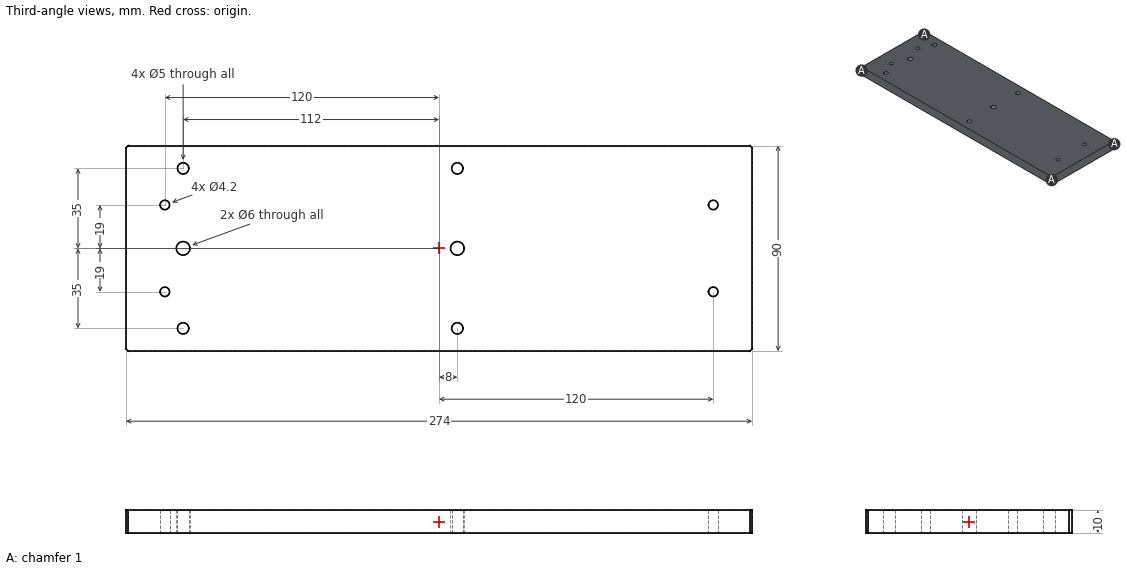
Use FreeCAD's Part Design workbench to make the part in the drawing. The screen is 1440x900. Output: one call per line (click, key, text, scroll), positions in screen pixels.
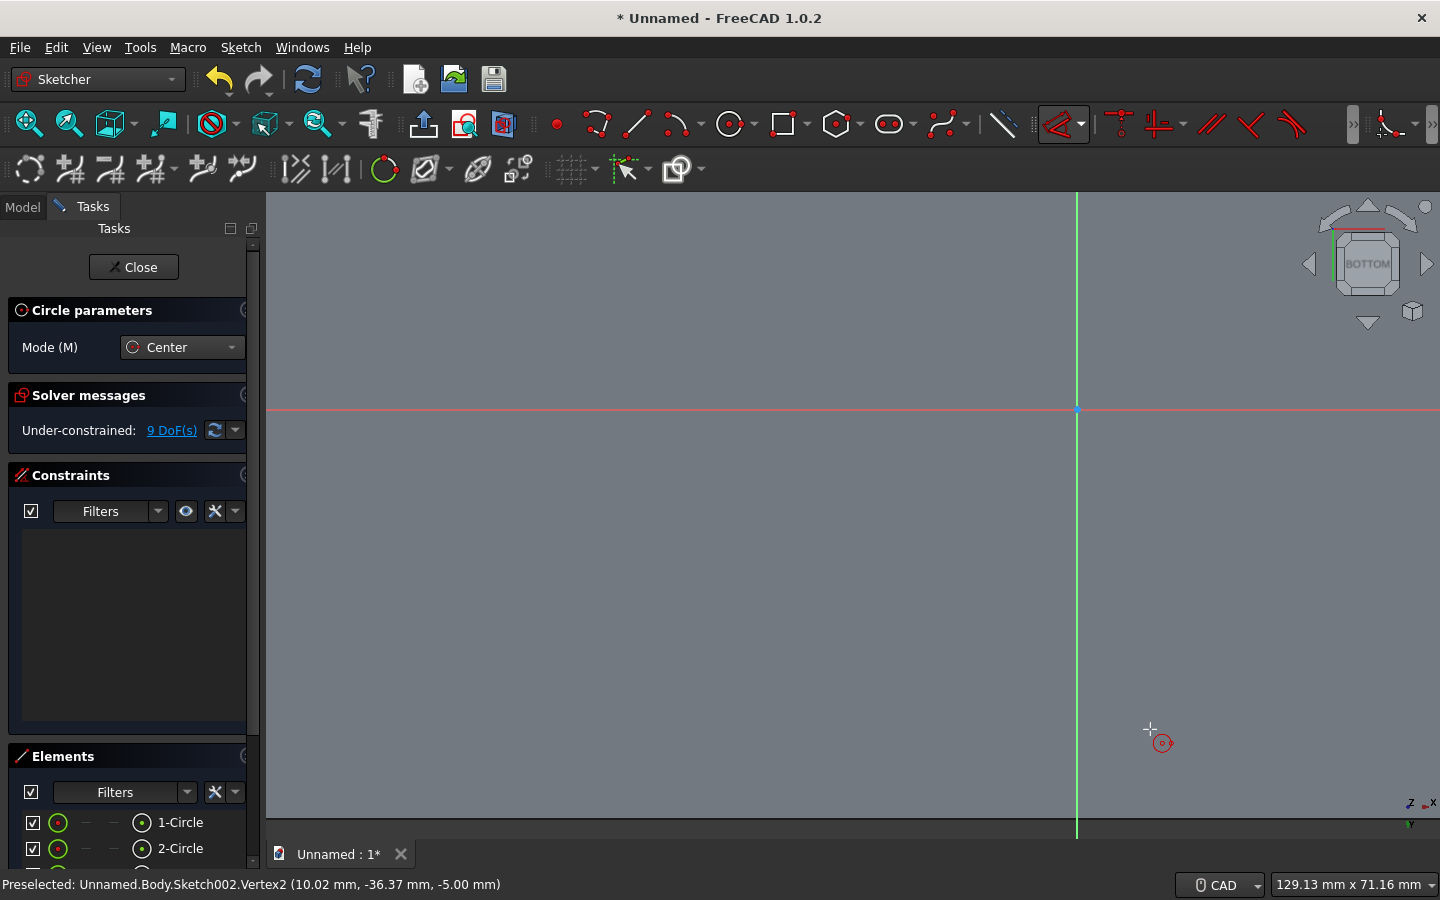
click(1150, 728)
click(1166, 712)
key(Escape)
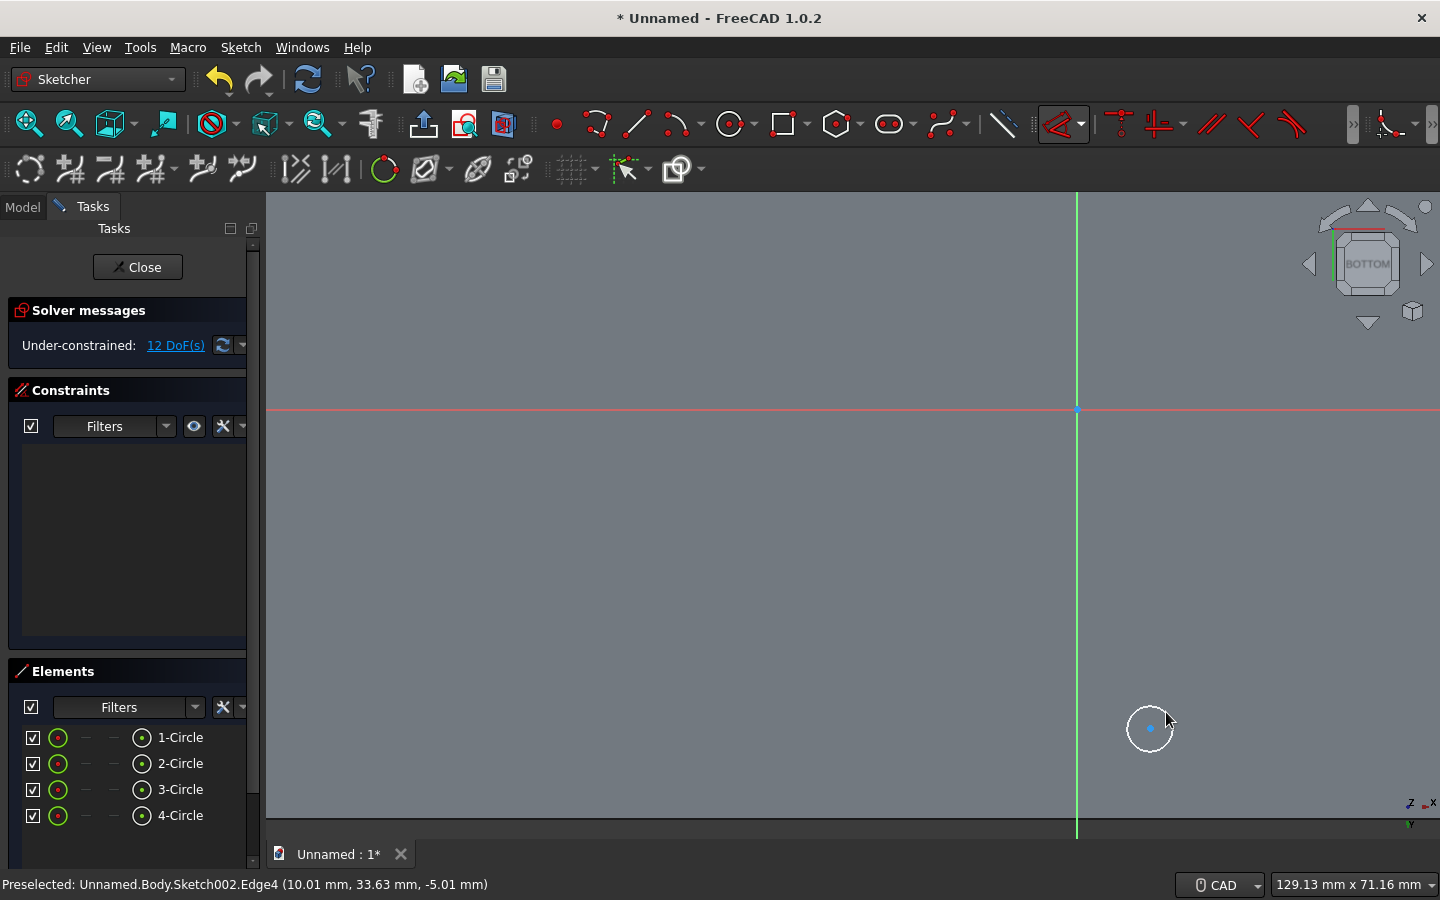
scroll(1150, 730, down, 2)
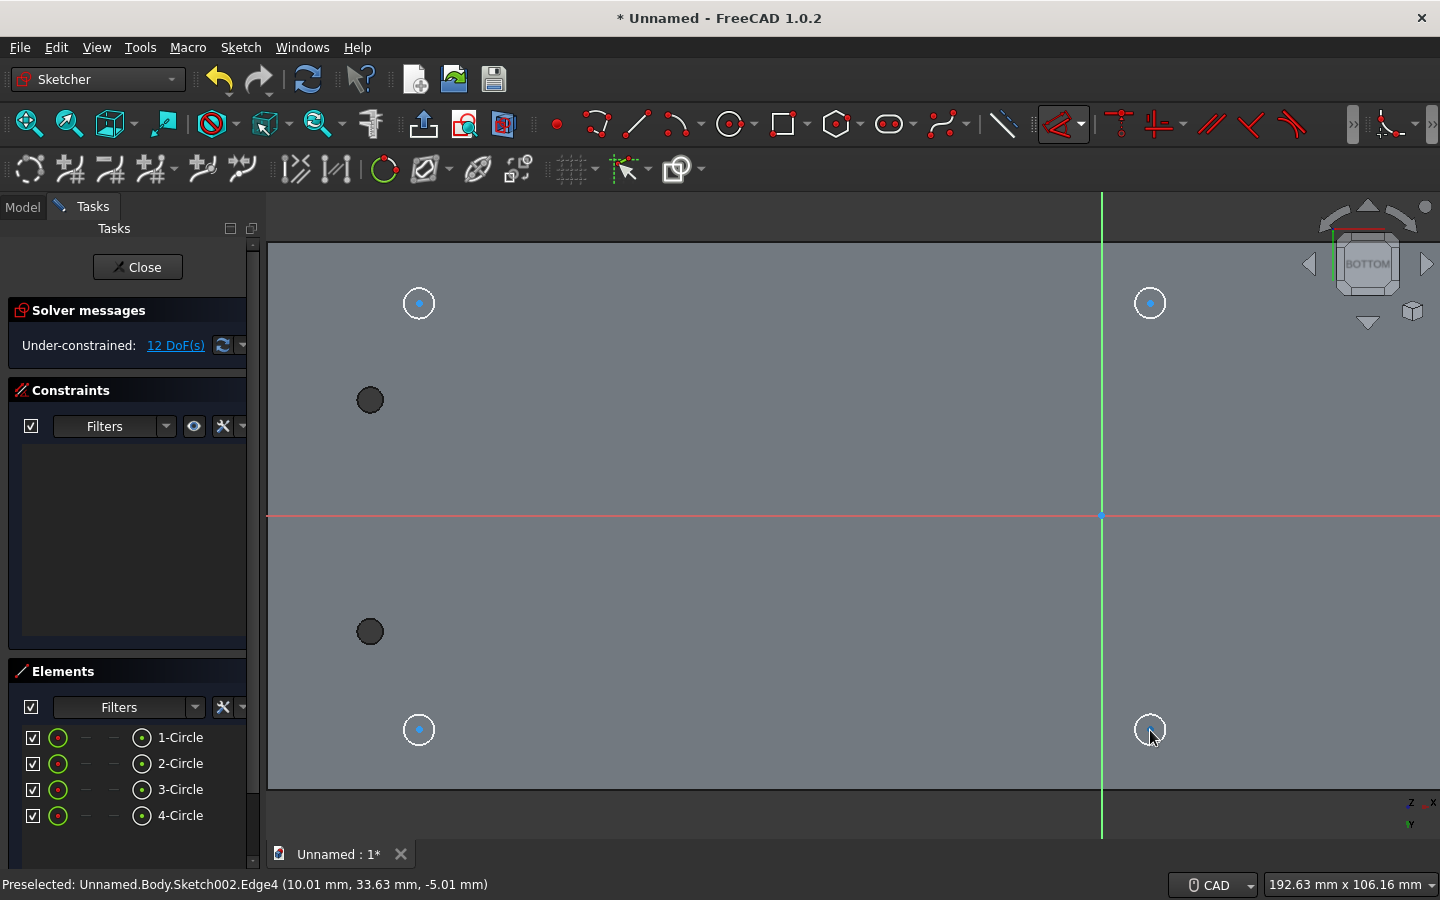
click(430, 719)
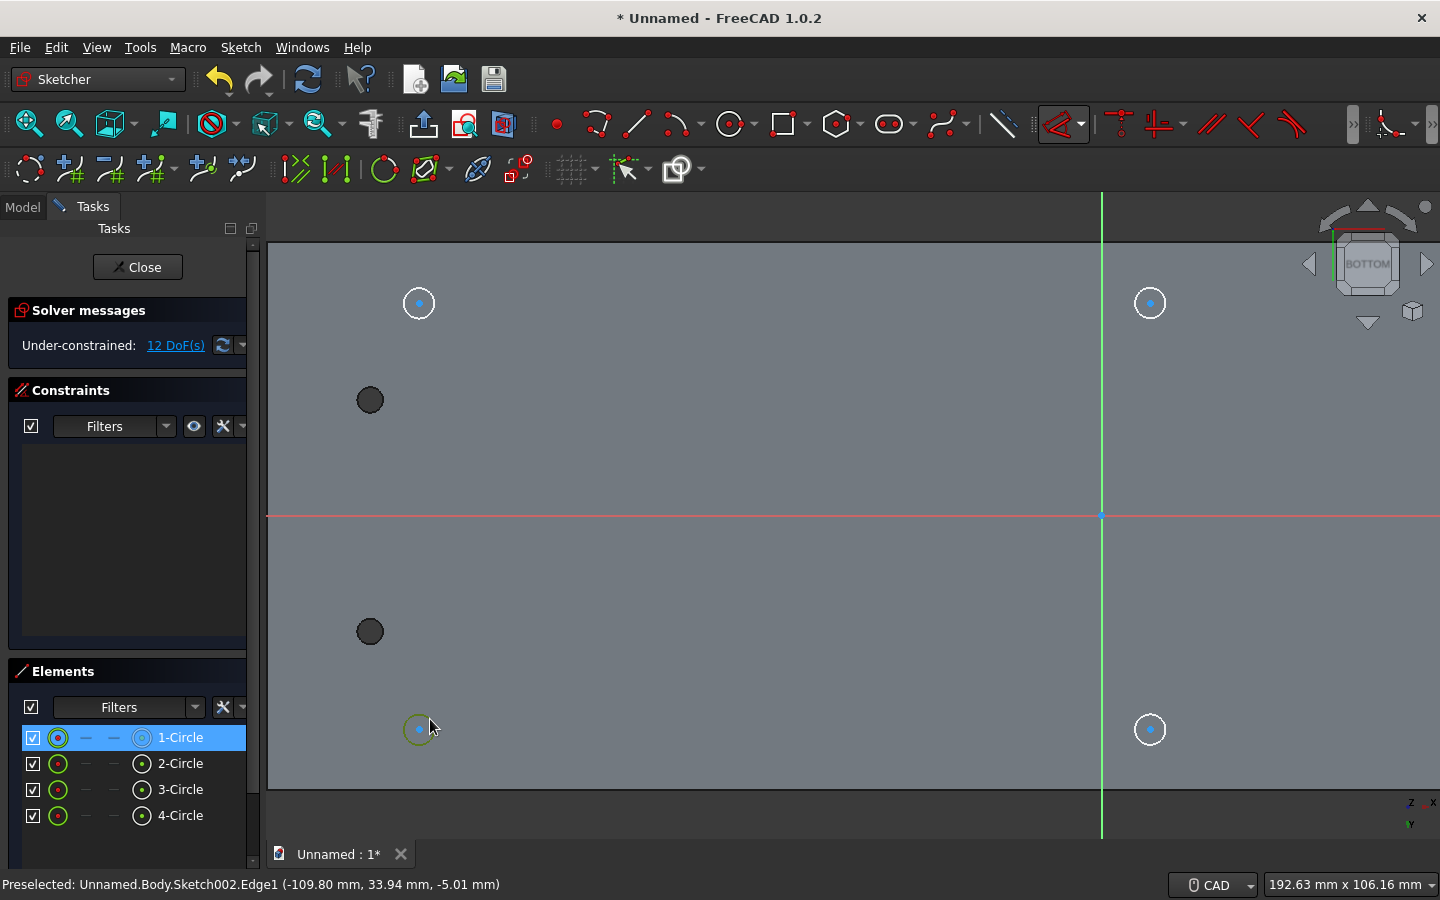
click(430, 293)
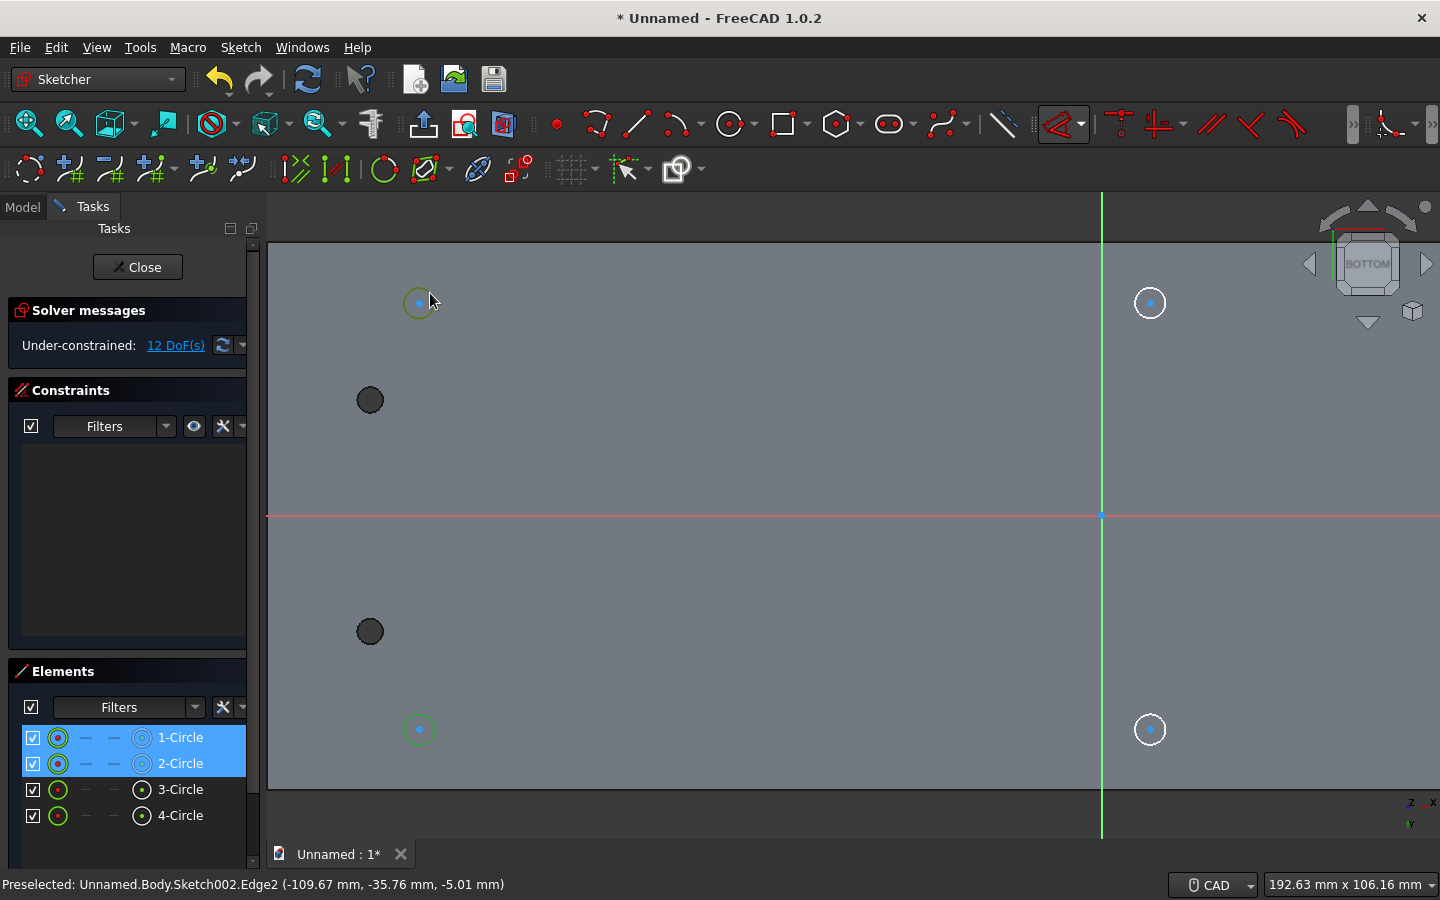
click(1161, 292)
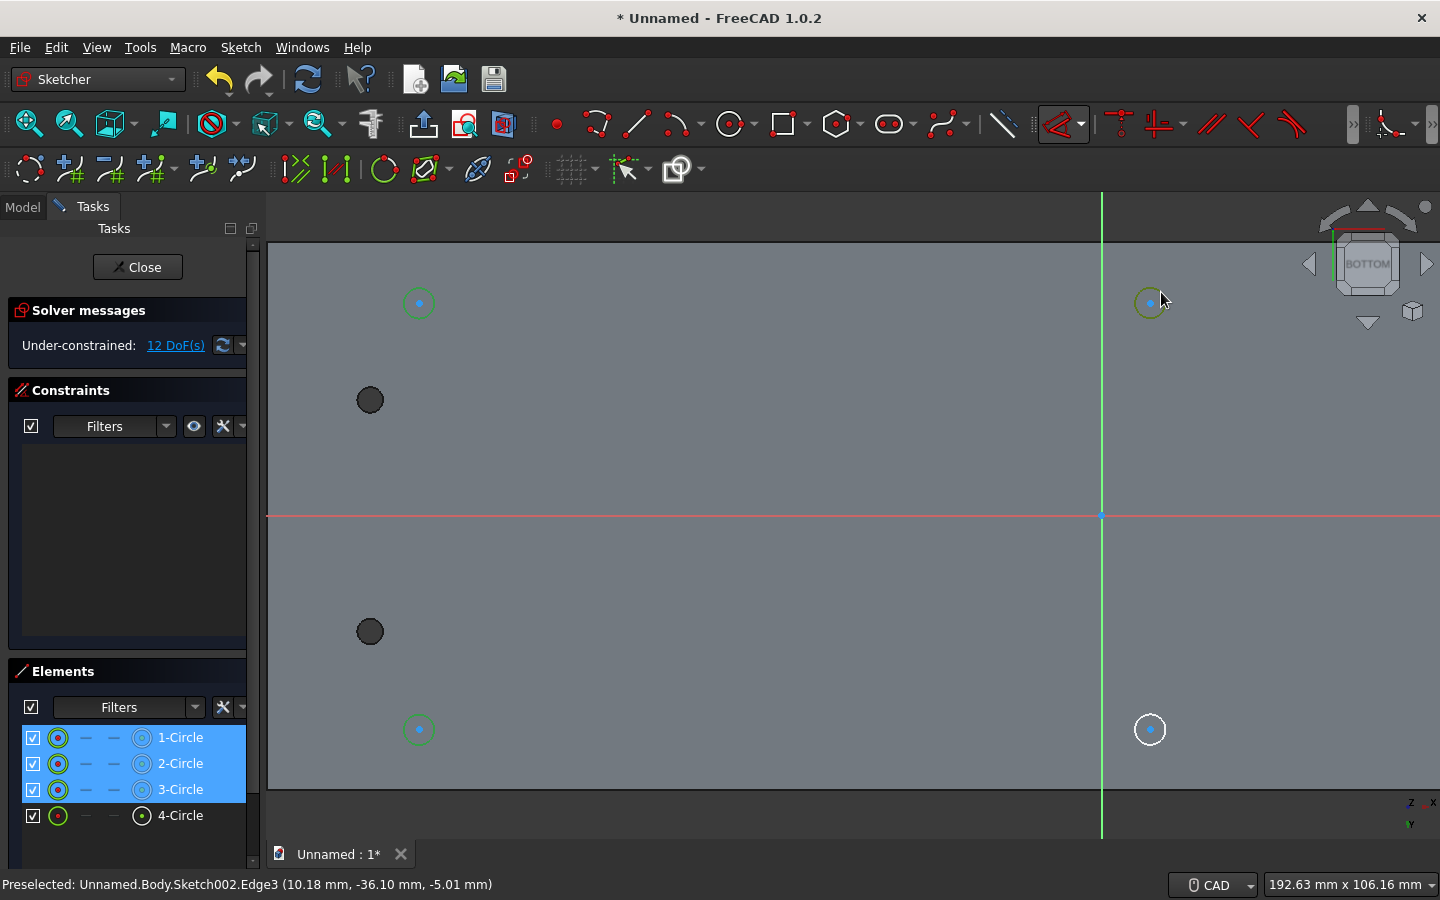
click(1161, 719)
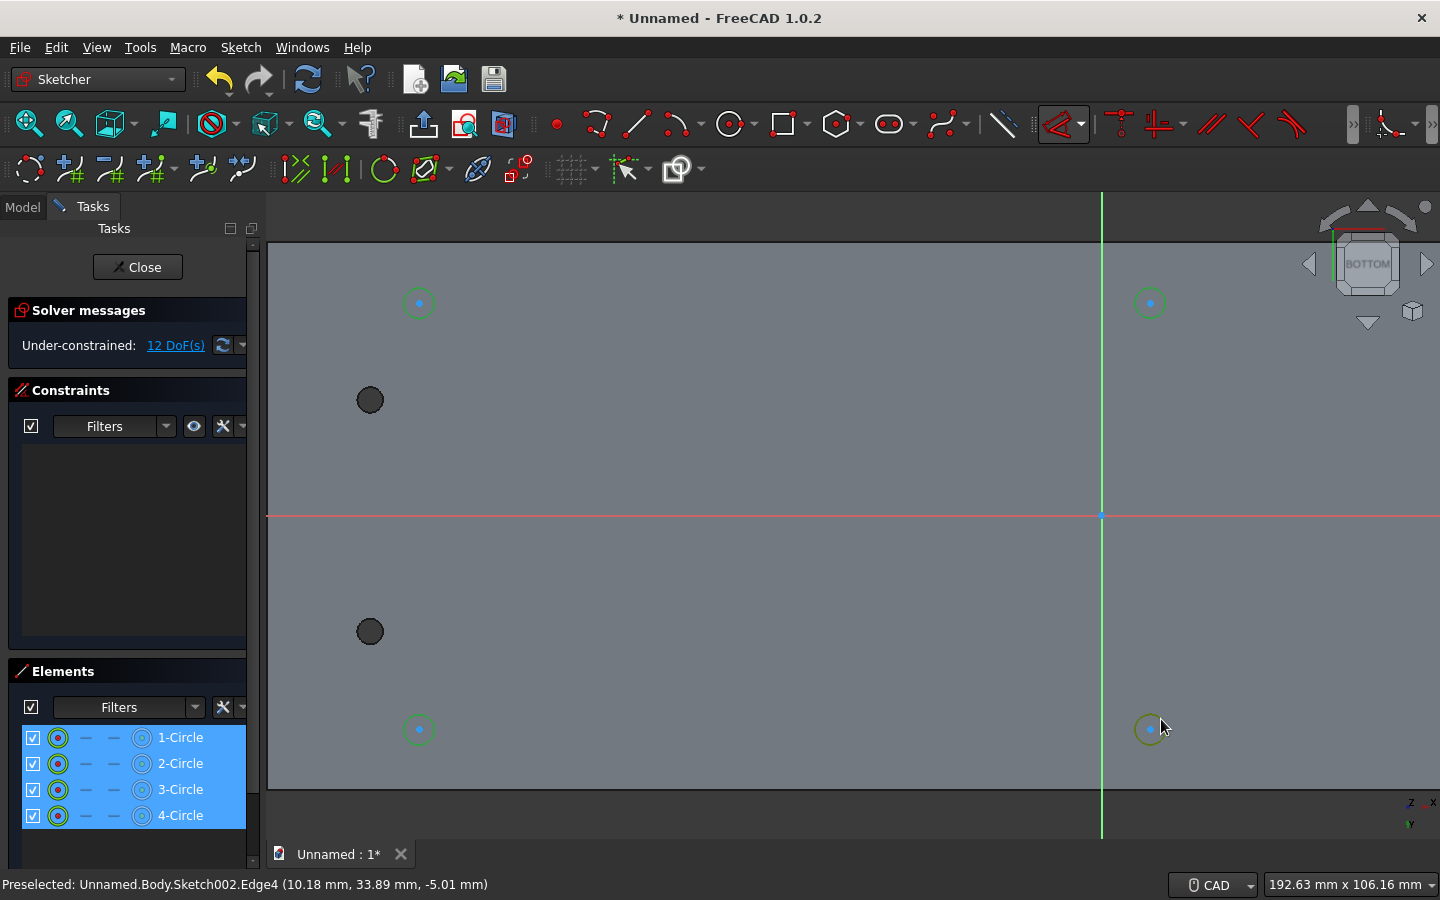
key(e)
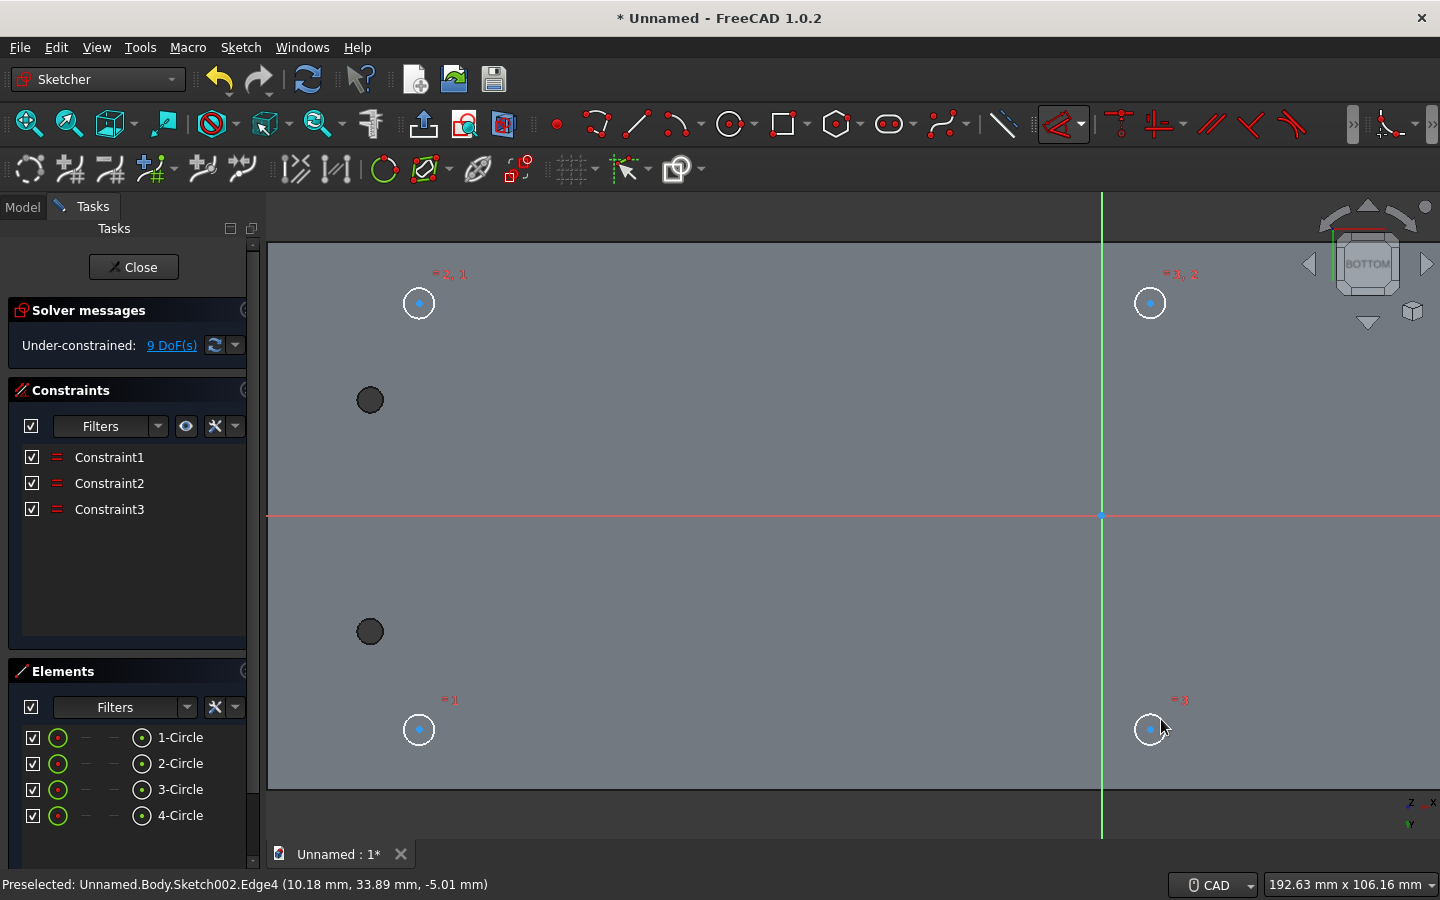
scroll(430, 719, up, 2)